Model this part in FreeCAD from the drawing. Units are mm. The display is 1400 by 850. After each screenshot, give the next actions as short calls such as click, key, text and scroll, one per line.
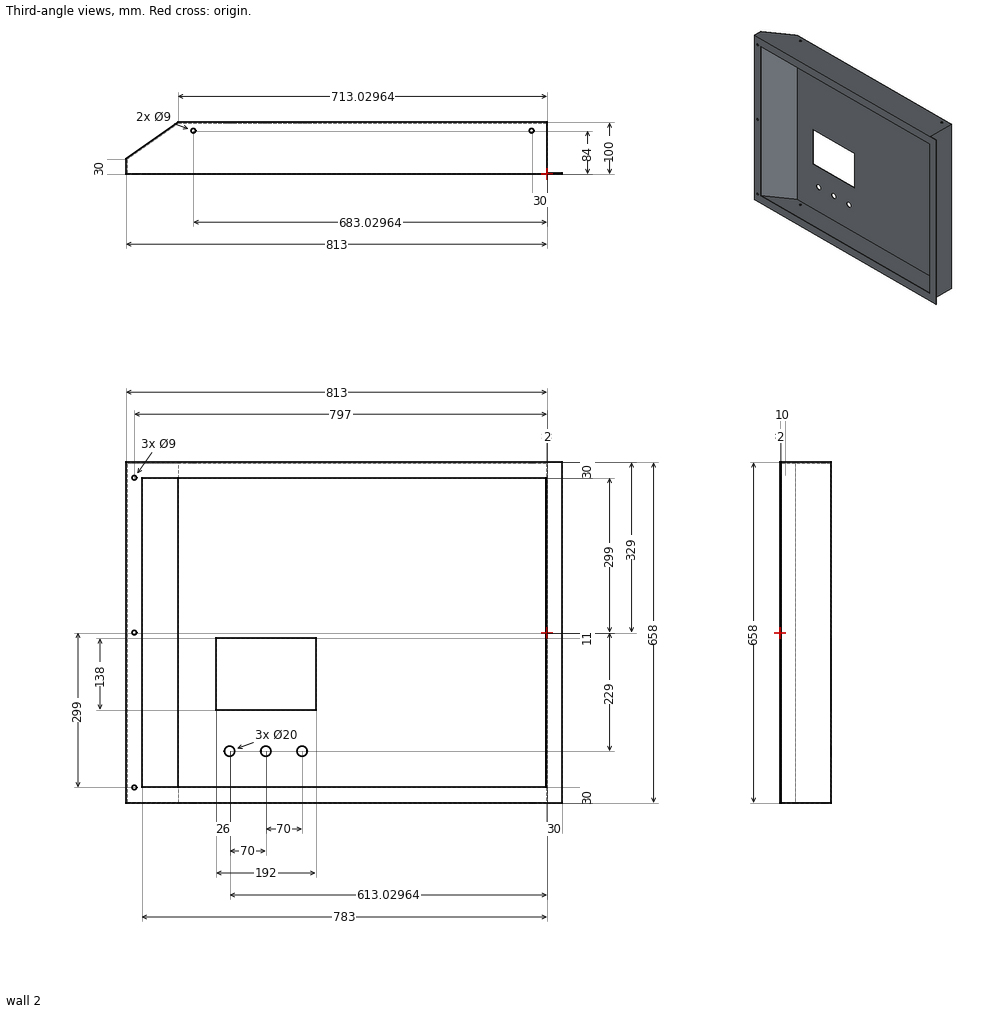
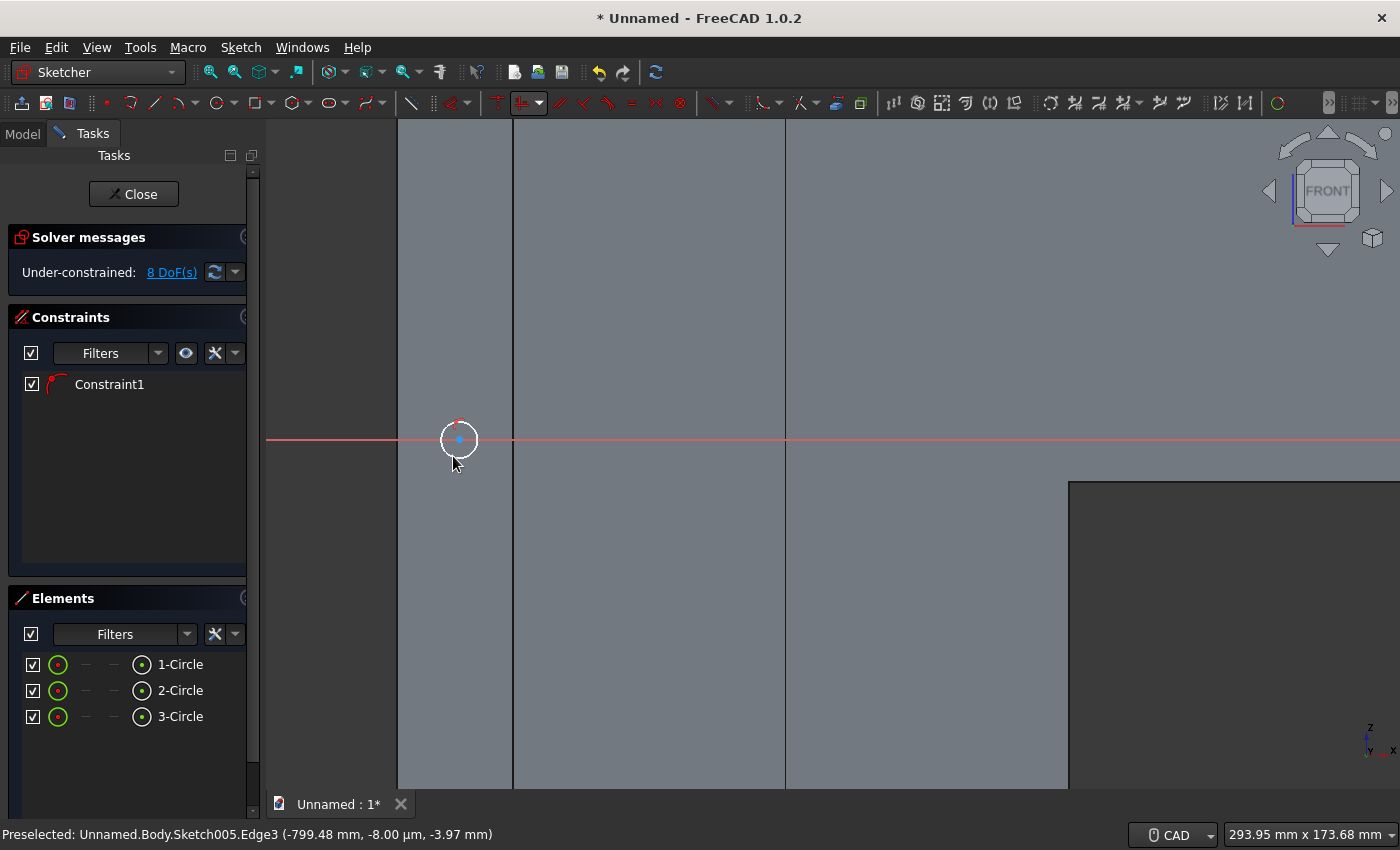
scroll(455, 458, down, 8)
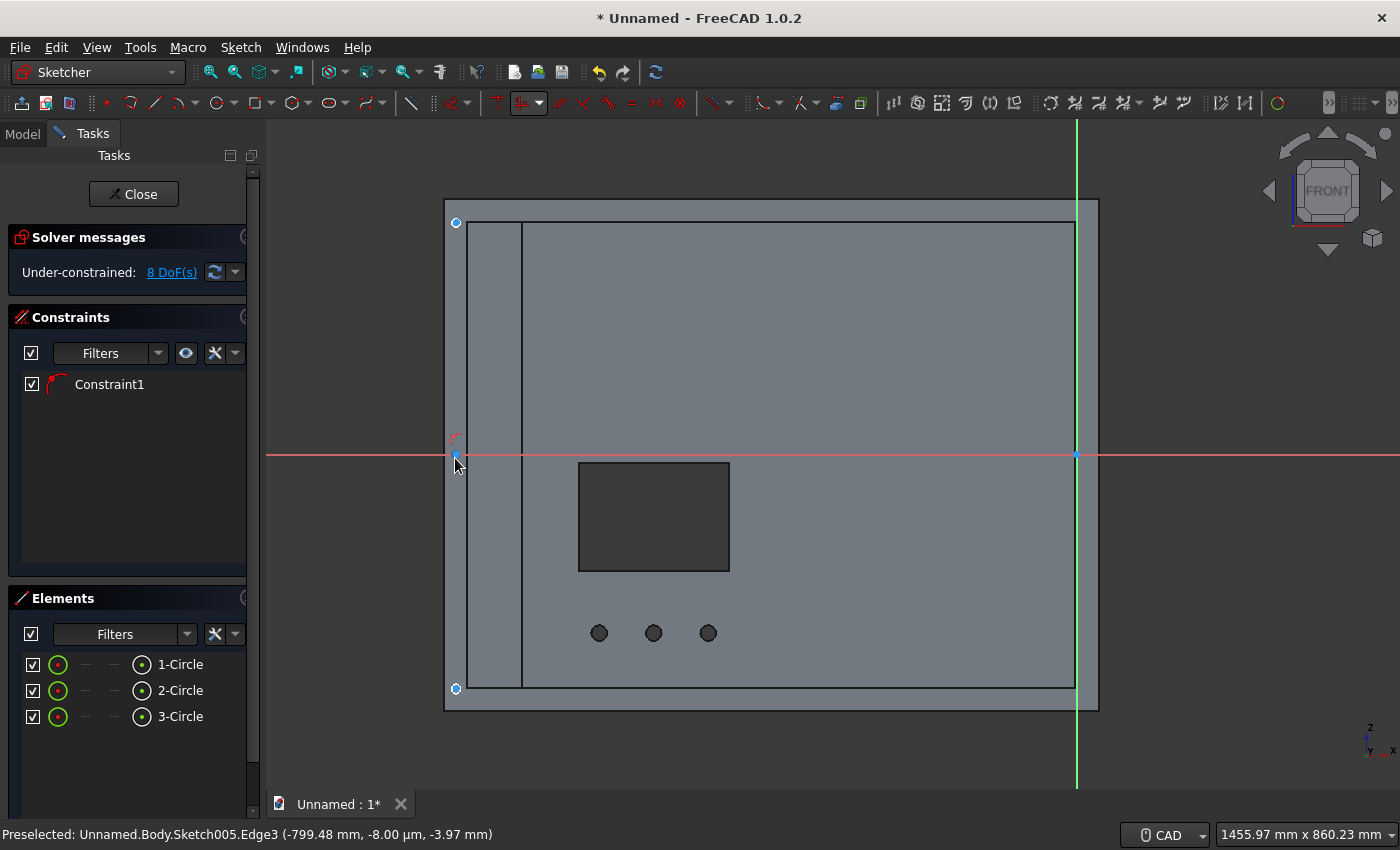
scroll(459, 220, up, 7)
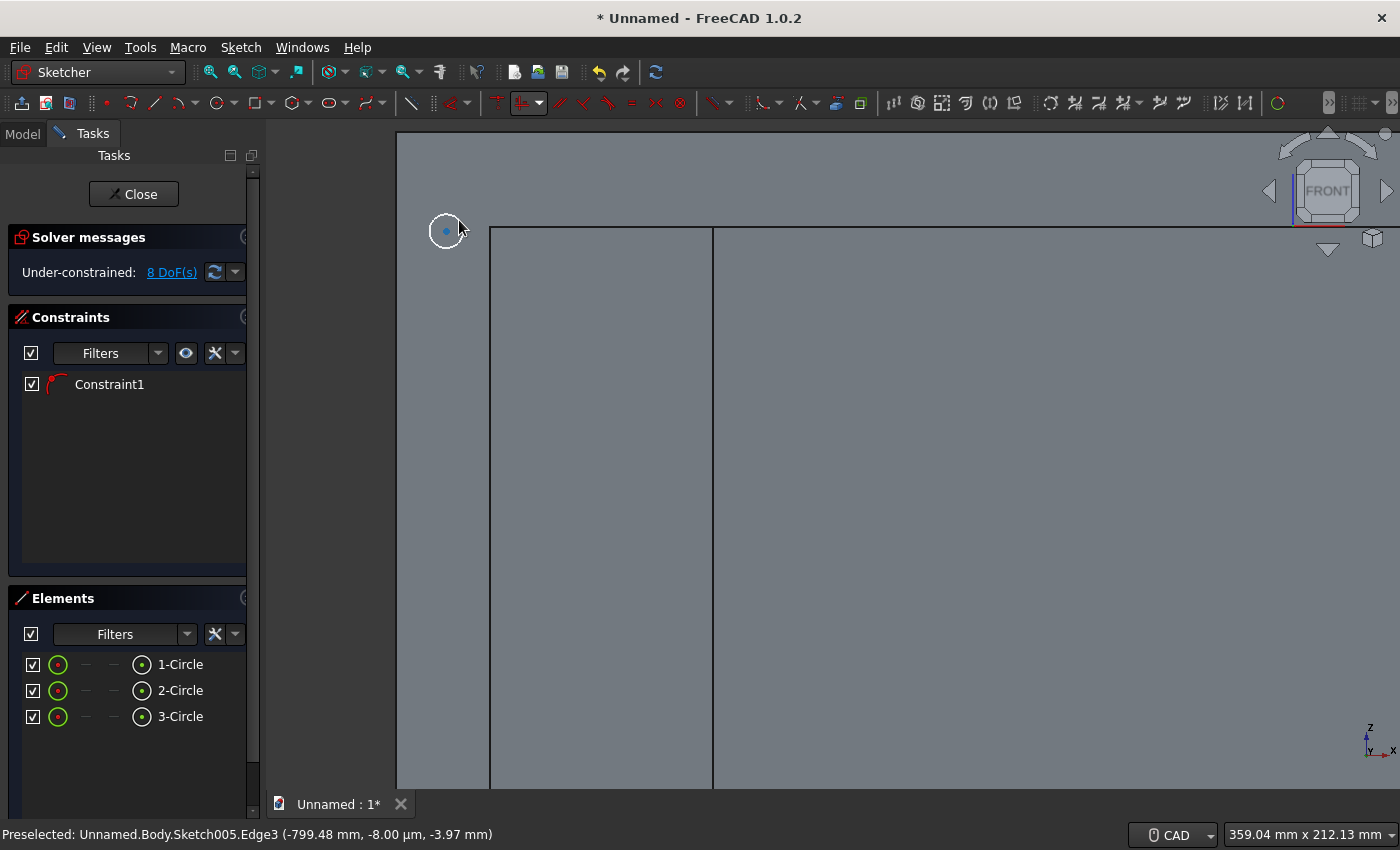
click(458, 219)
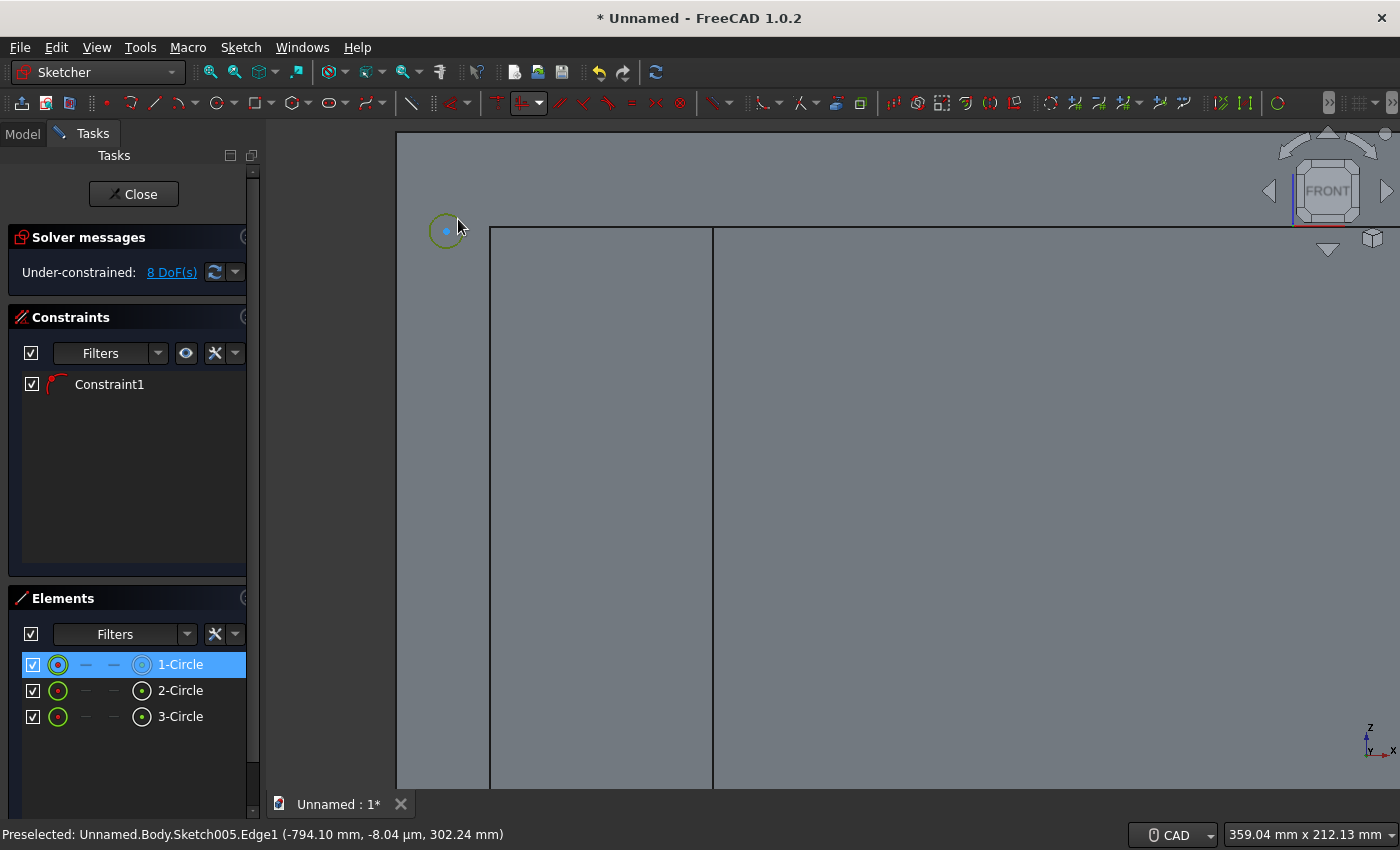
scroll(459, 219, down, 7)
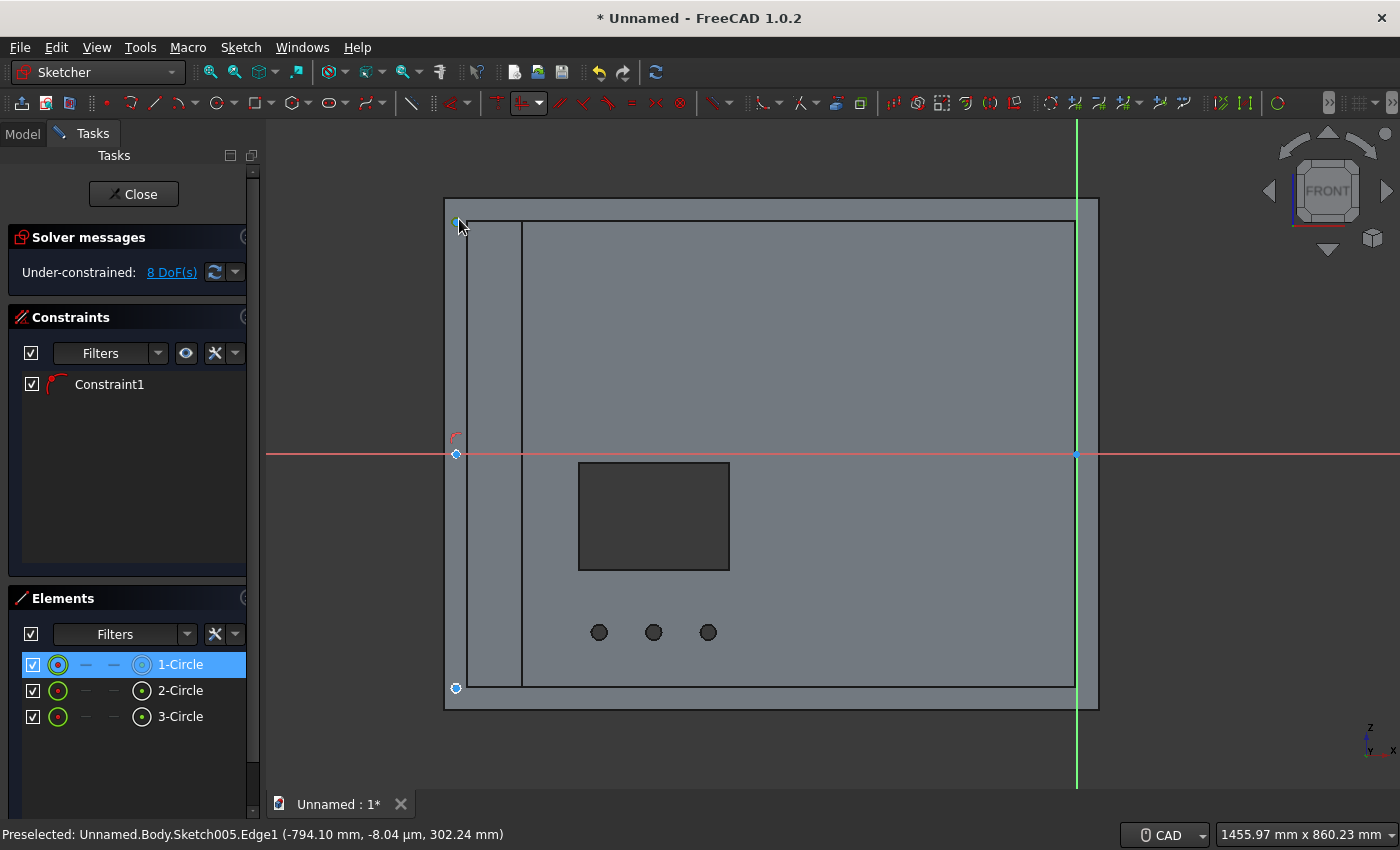
scroll(459, 685, up, 6)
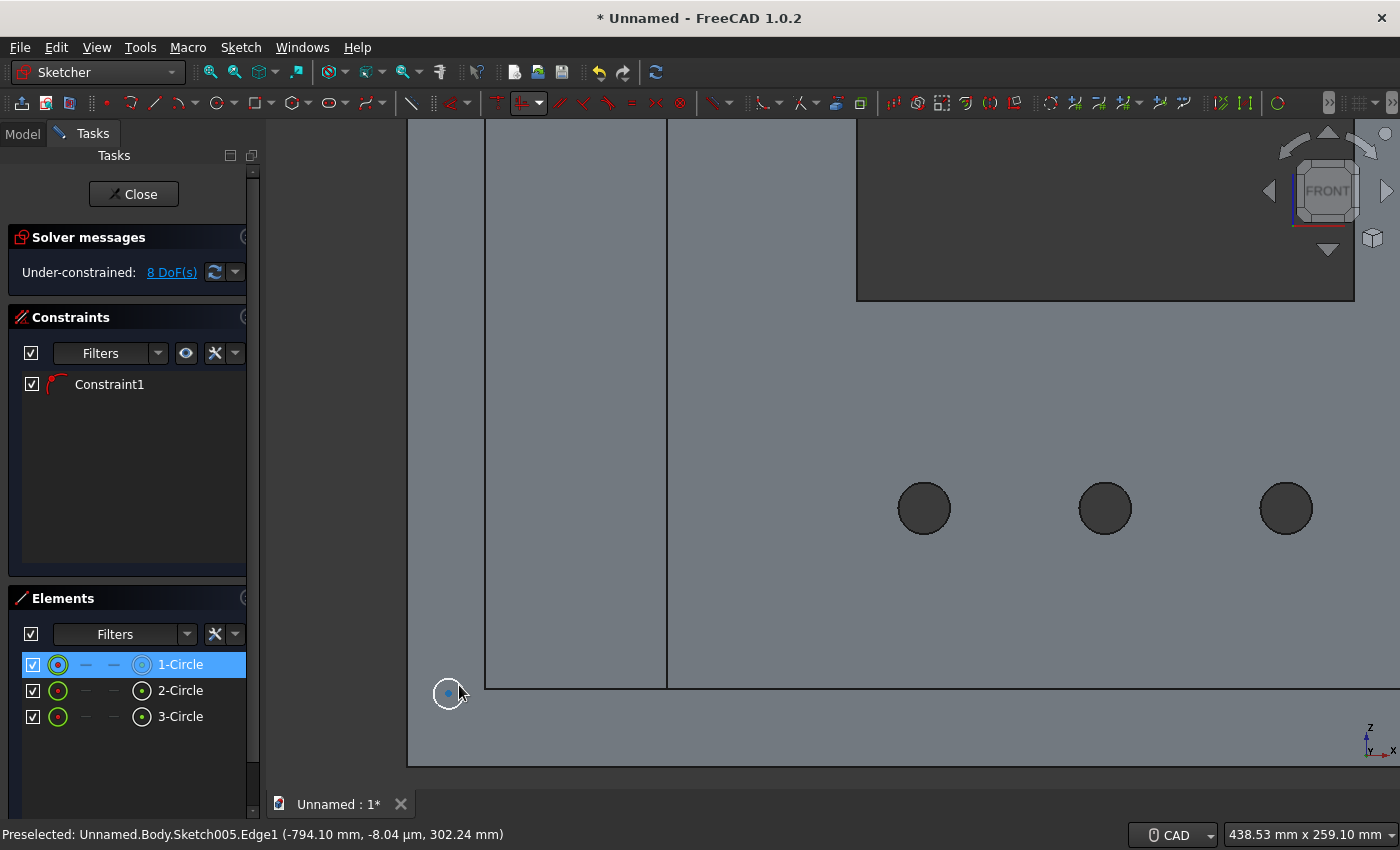
click(459, 683)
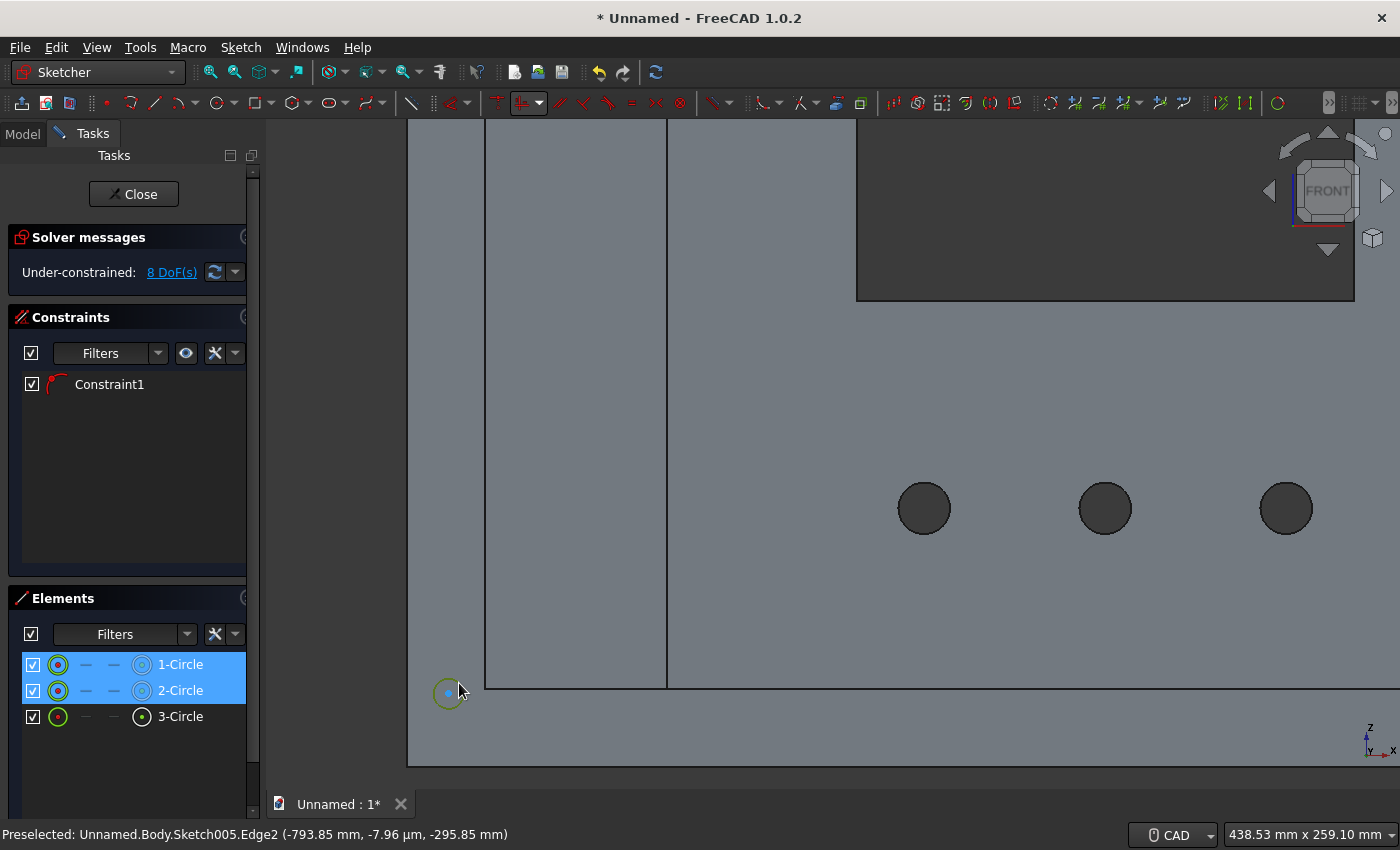
scroll(459, 686, down, 6)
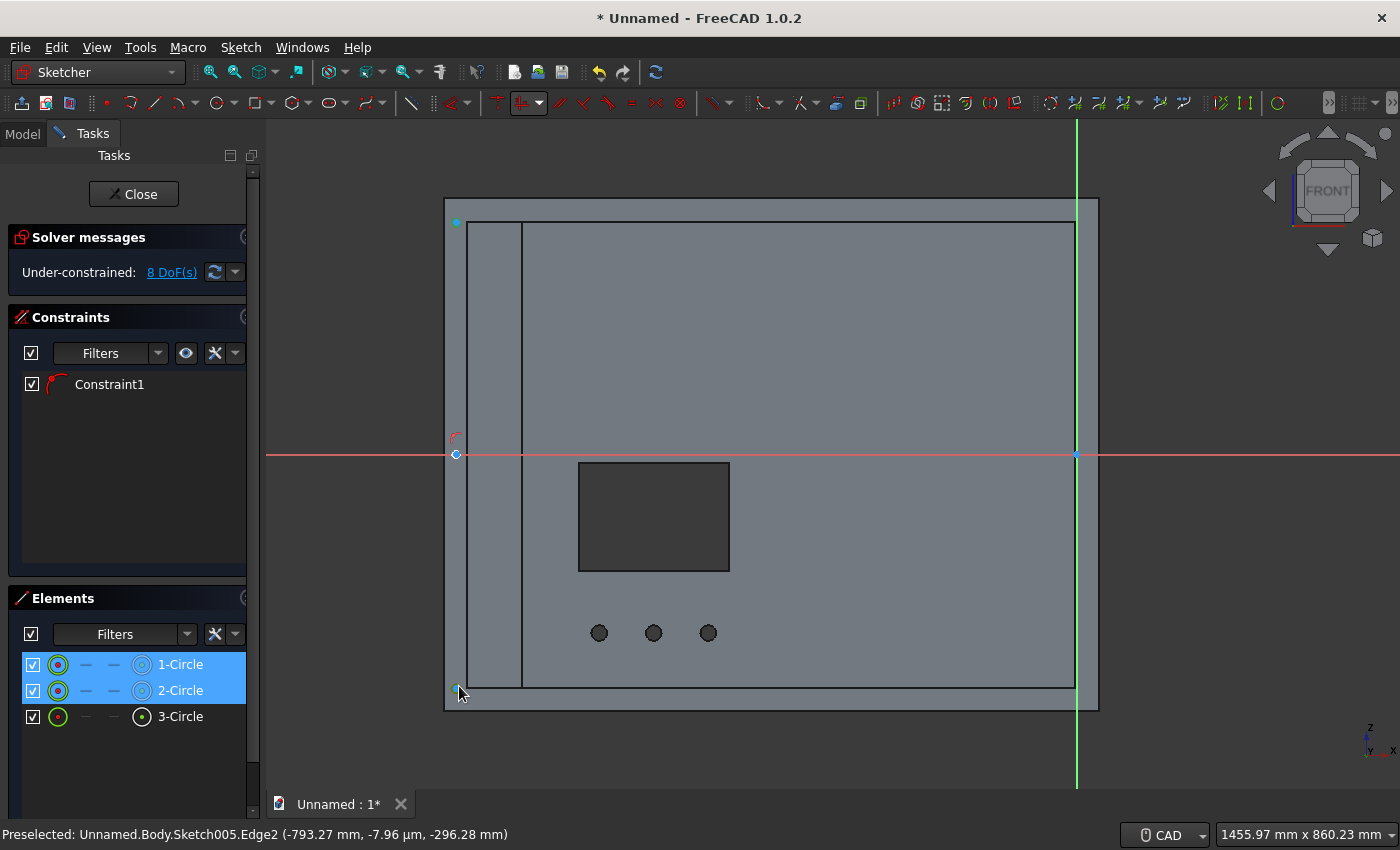
scroll(456, 451, up, 7)